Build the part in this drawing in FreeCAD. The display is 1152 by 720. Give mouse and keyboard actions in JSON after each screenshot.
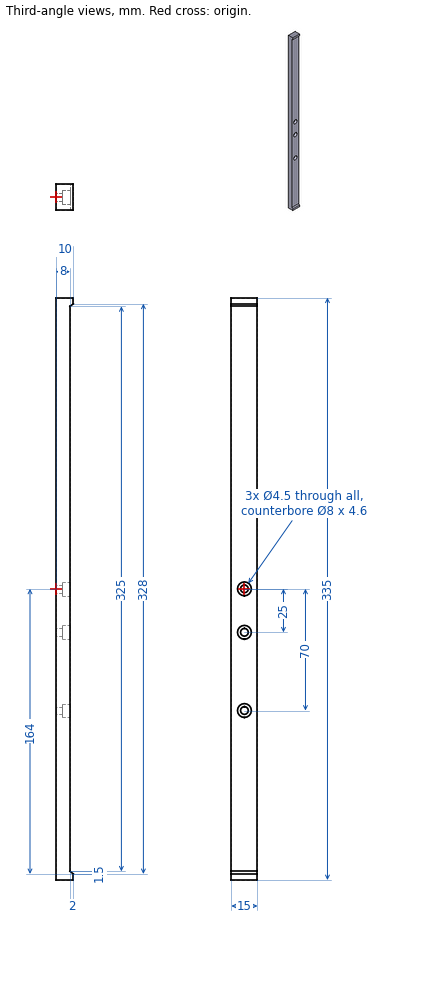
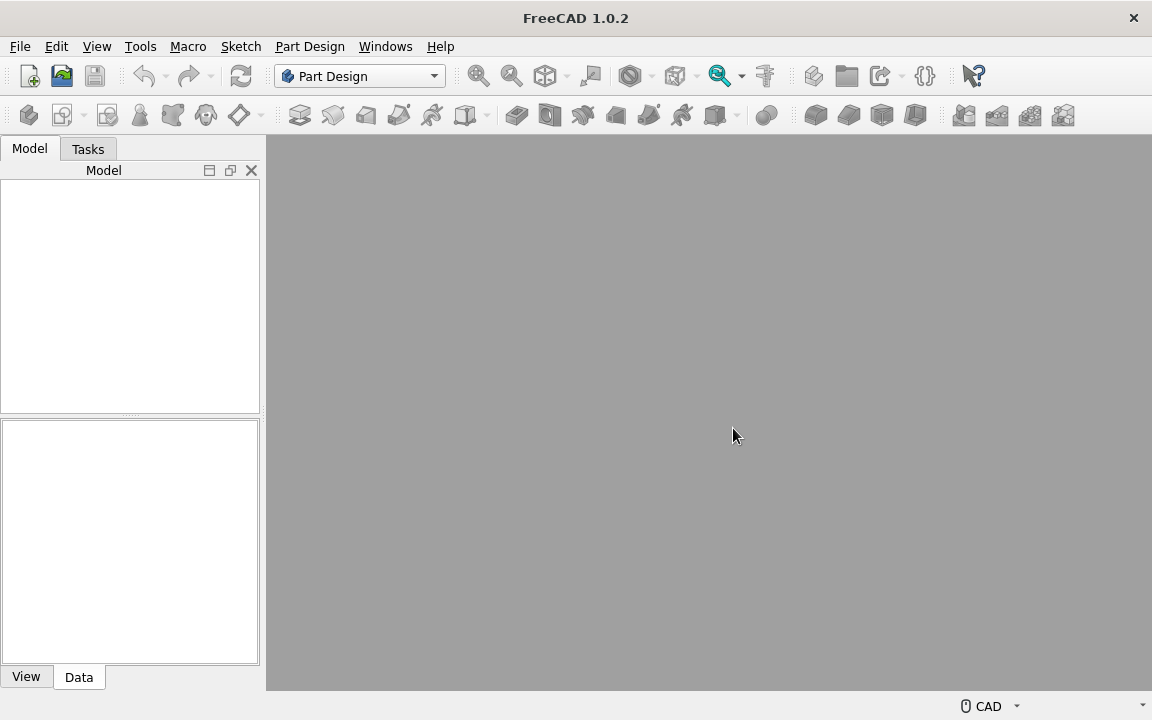
{"action": "key", "text": "ctrl+n"}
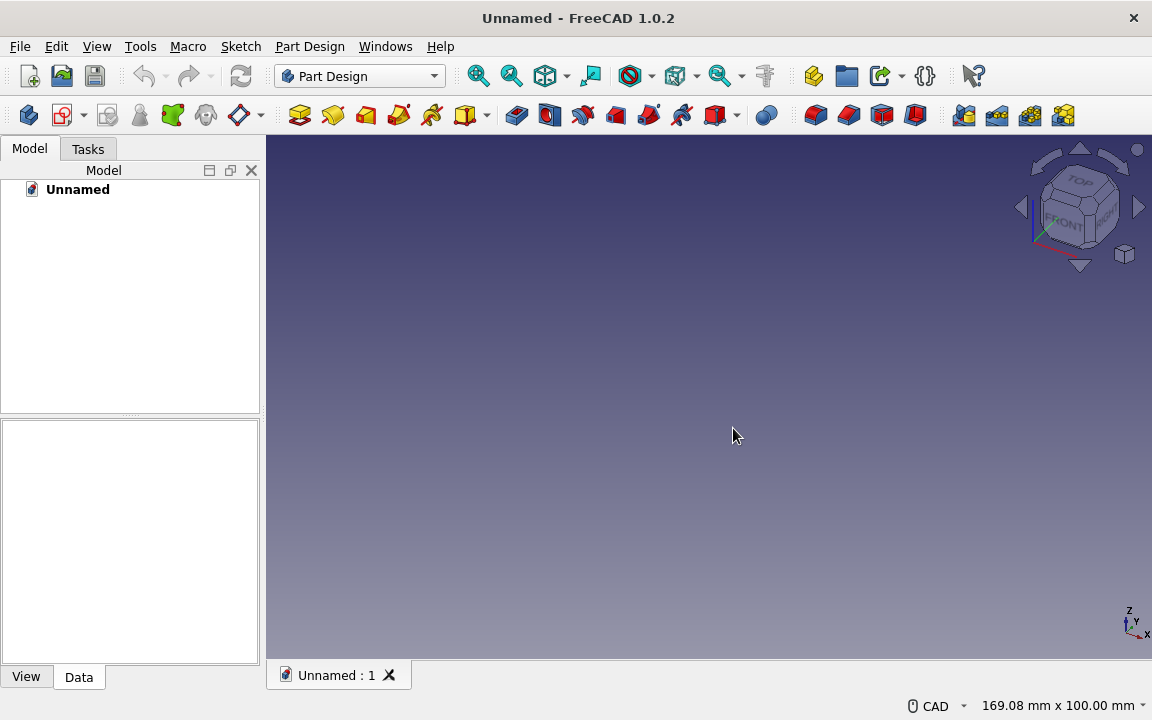
{"action": "left_click", "coordinate": [62, 116]}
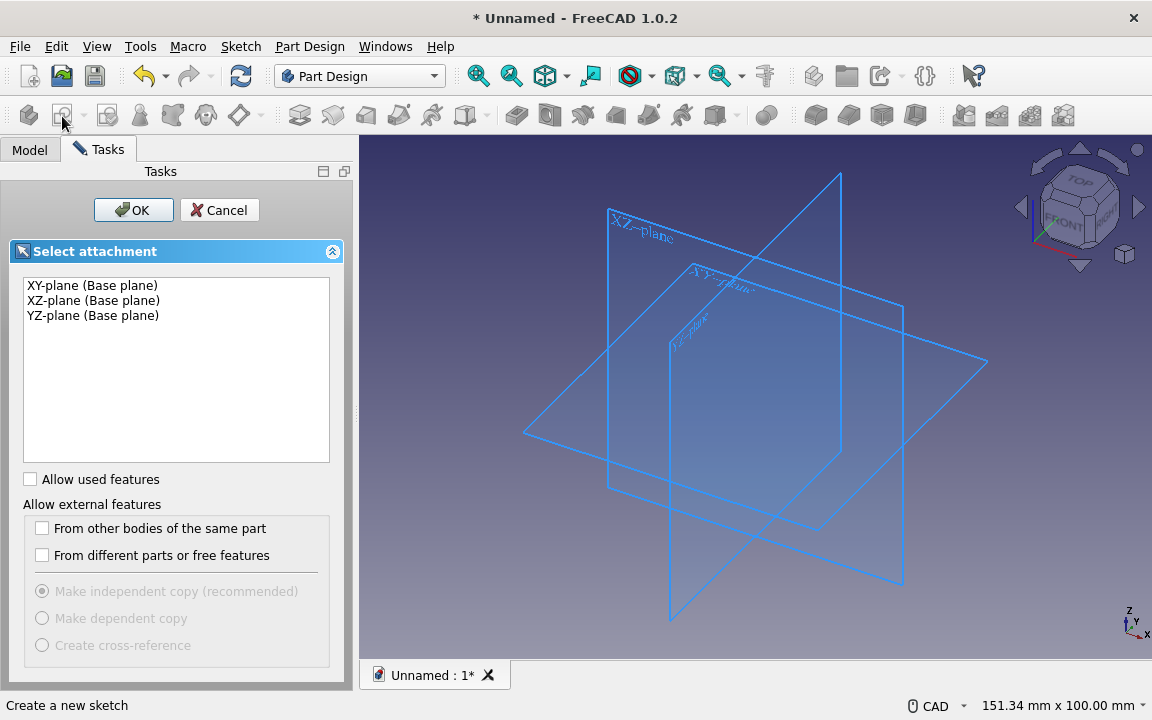
{"action": "left_click", "coordinate": [84, 316]}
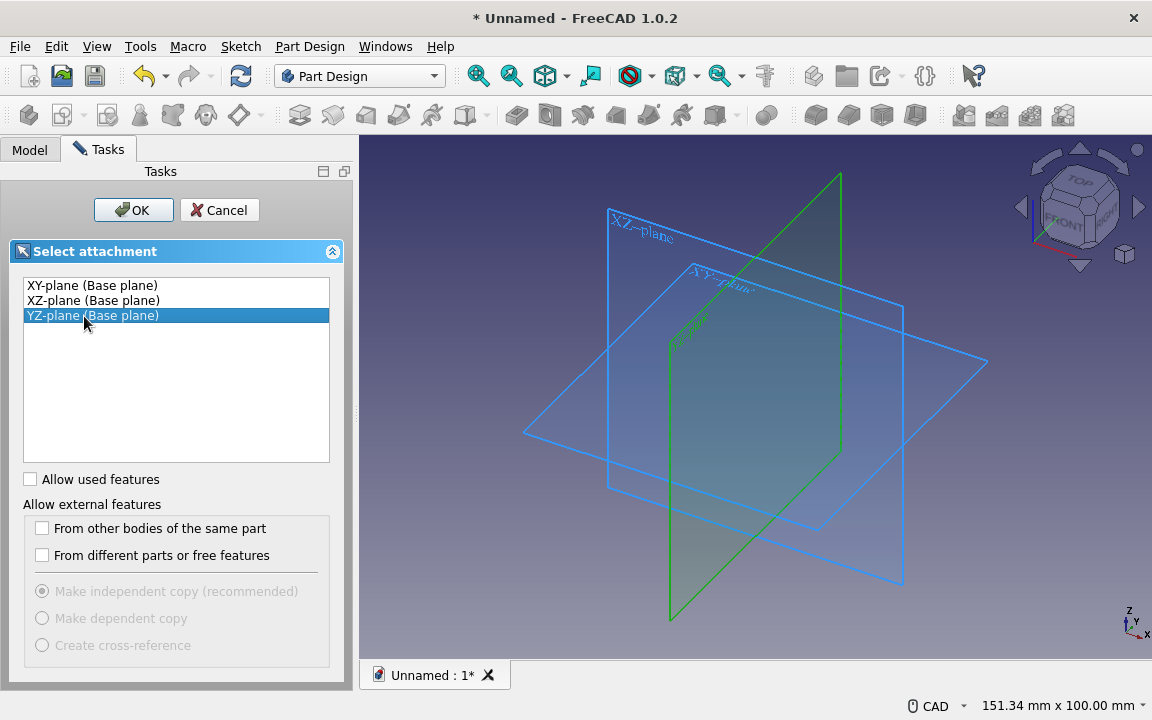
{"action": "left_click", "coordinate": [134, 210]}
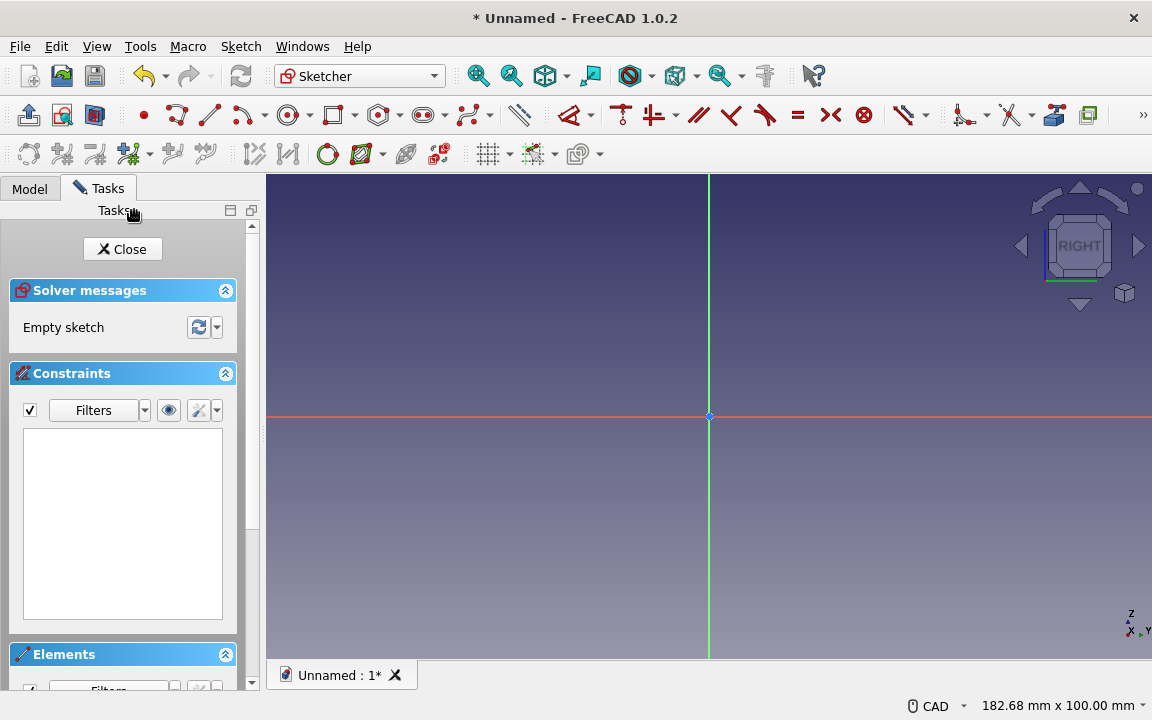
{"action": "scroll", "coordinate": [623, 416], "scroll_direction": "down", "scroll_amount": 8}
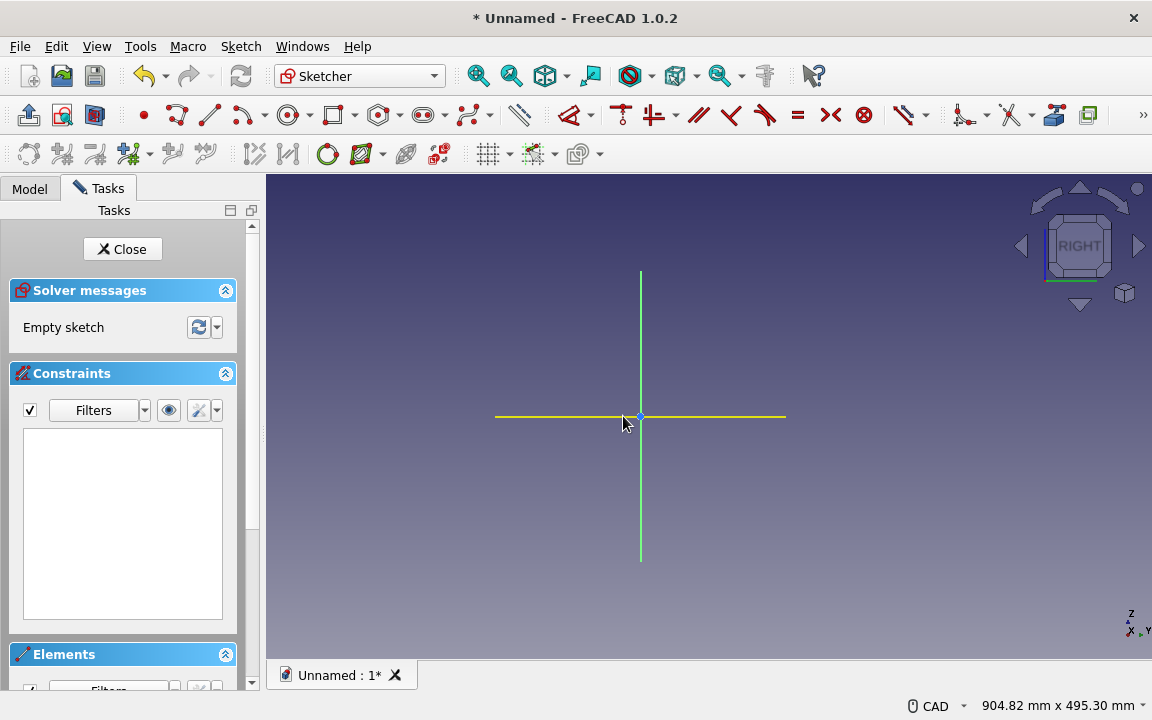
{"action": "key", "text": "g v"}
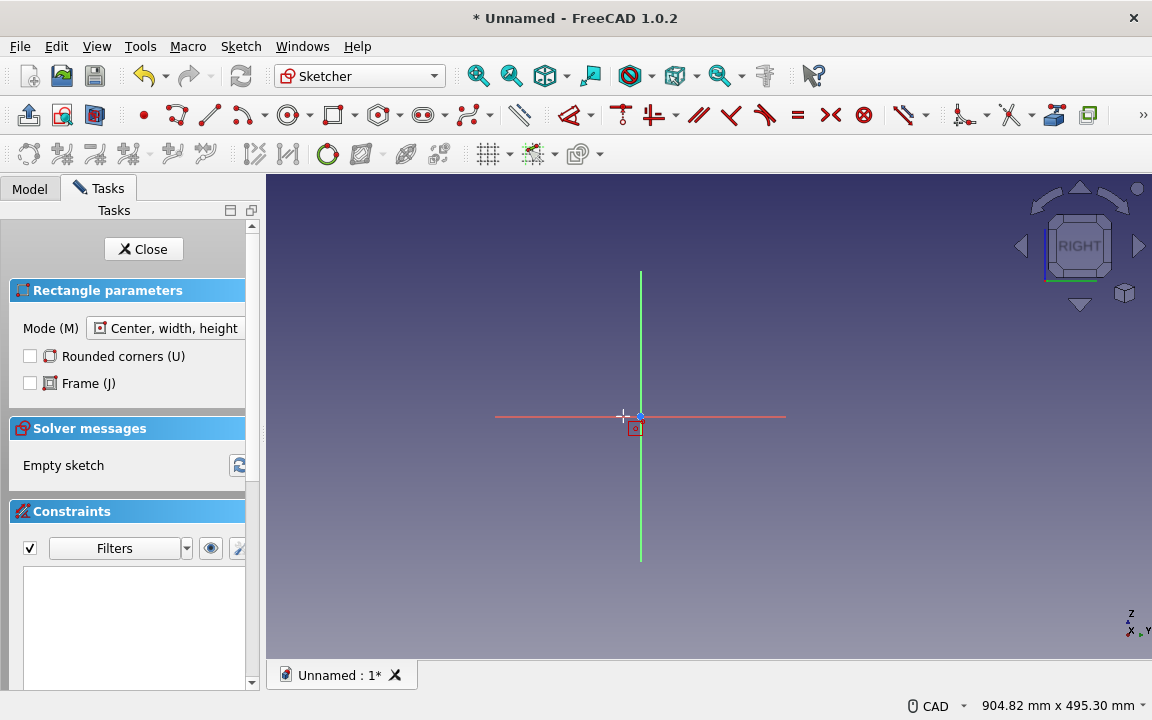
{"action": "scroll", "coordinate": [641, 416], "scroll_direction": "up", "scroll_amount": 4}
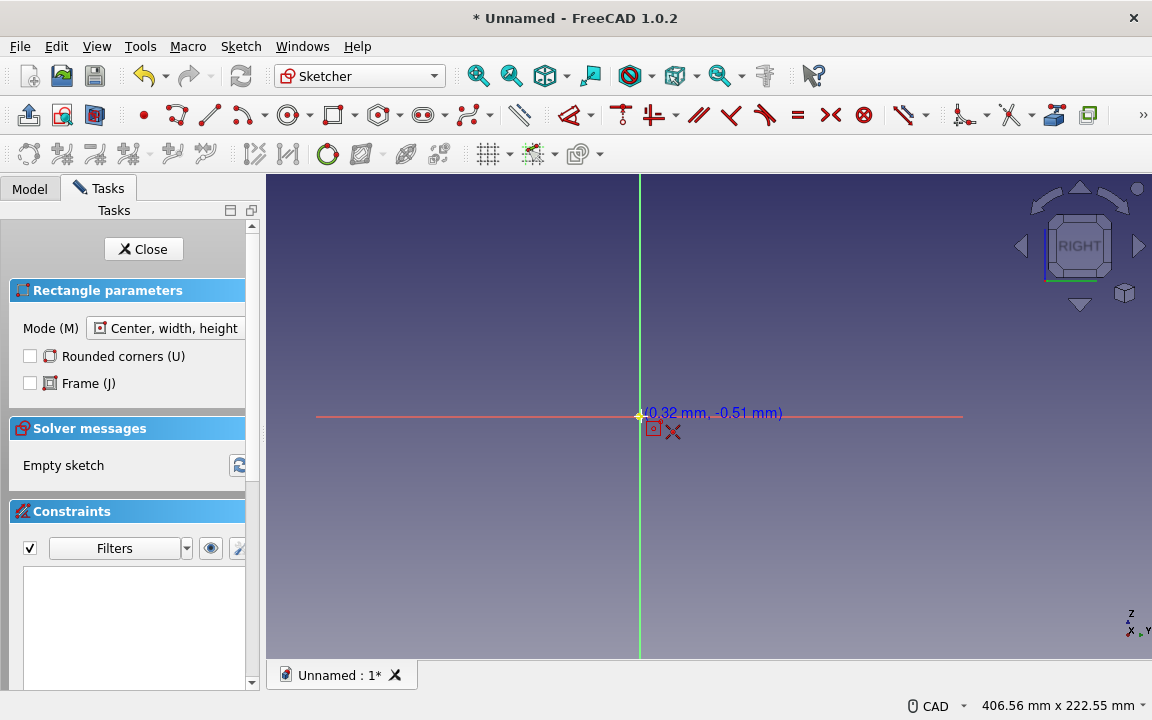
{"action": "left_click", "coordinate": [640, 416]}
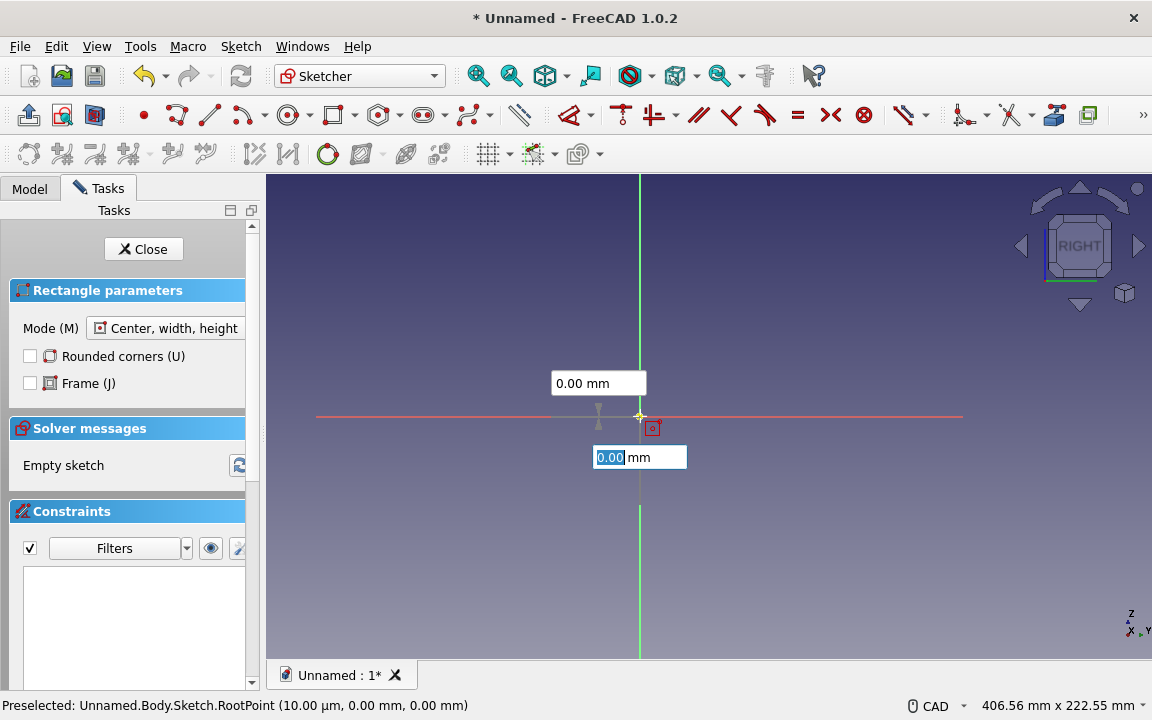
{"action": "scroll", "coordinate": [641, 416], "scroll_direction": "down", "scroll_amount": 4}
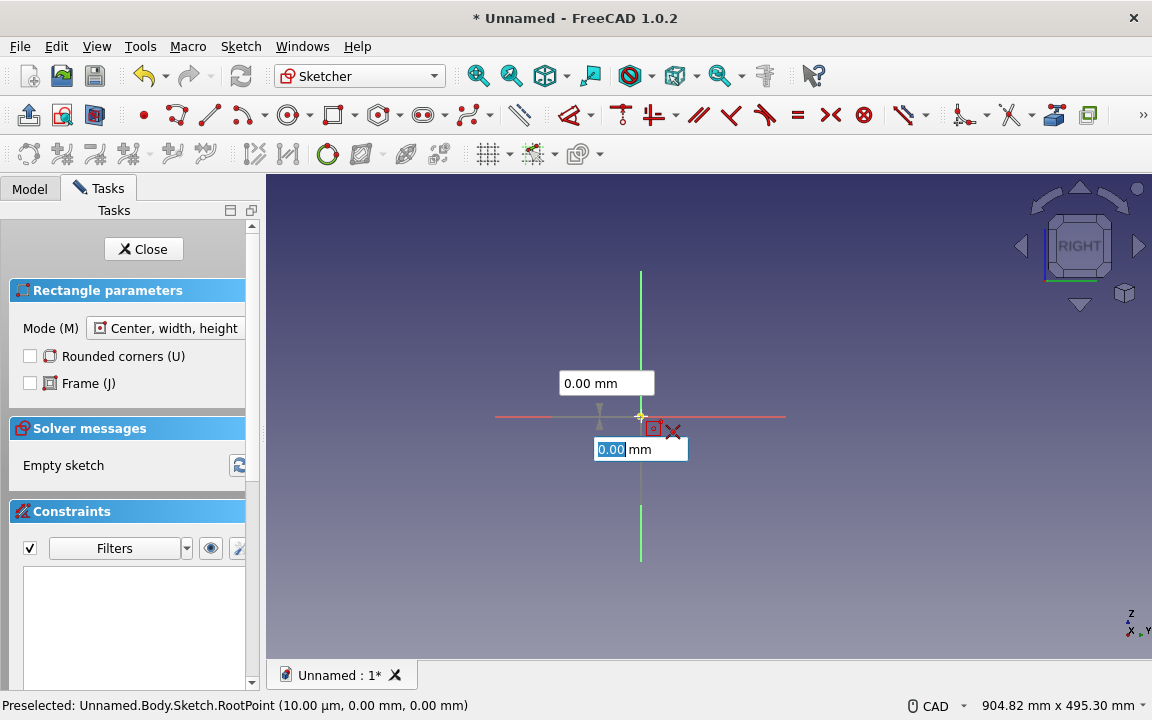
{"action": "scroll", "coordinate": [648, 252], "scroll_direction": "up", "scroll_amount": 4}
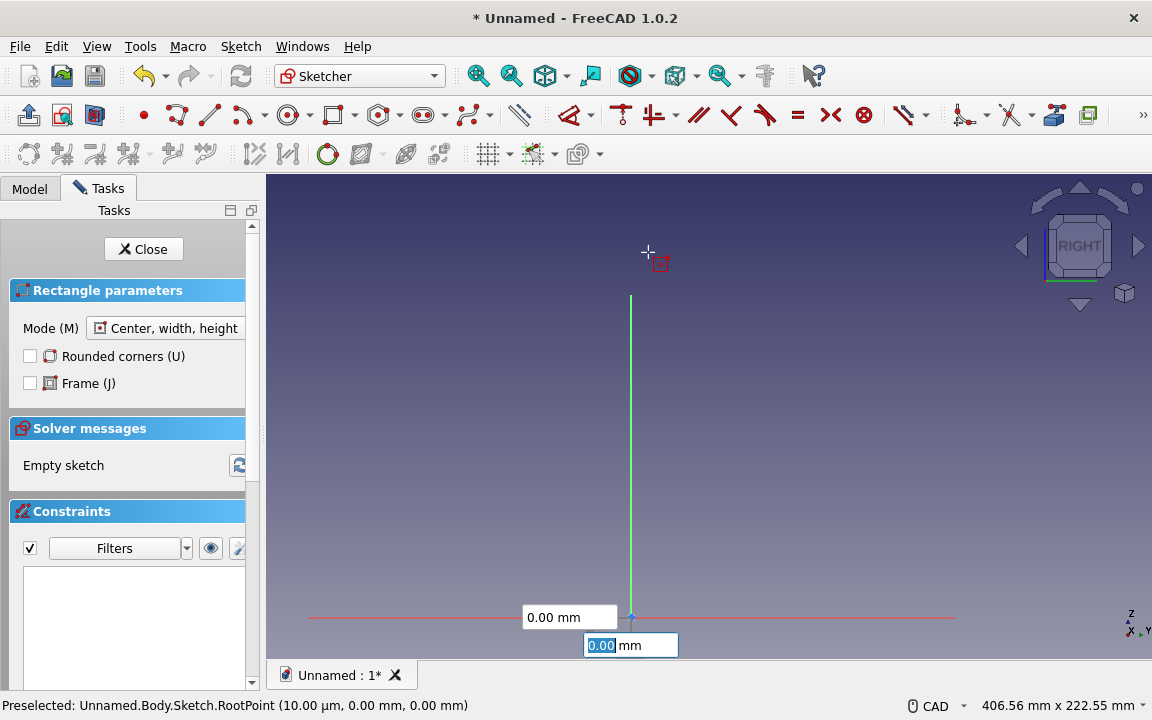
{"action": "left_click", "coordinate": [648, 253]}
{"action": "key", "text": "Escape"}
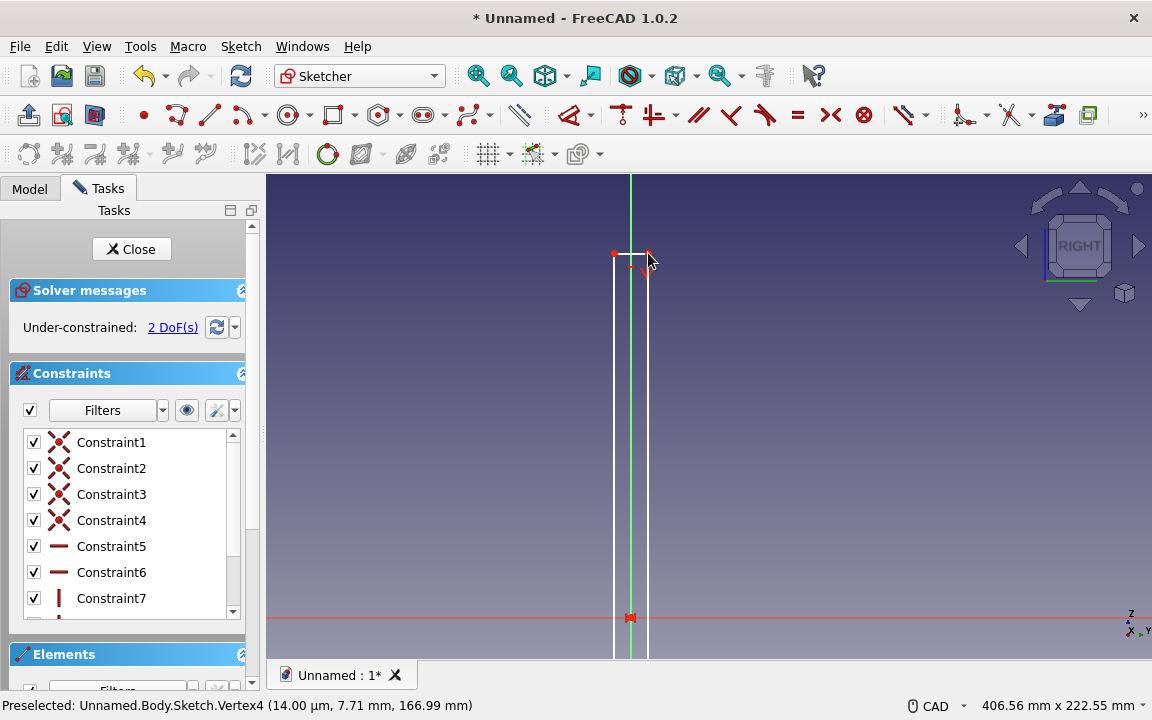
{"action": "scroll", "coordinate": [648, 252], "scroll_direction": "down", "scroll_amount": 4}